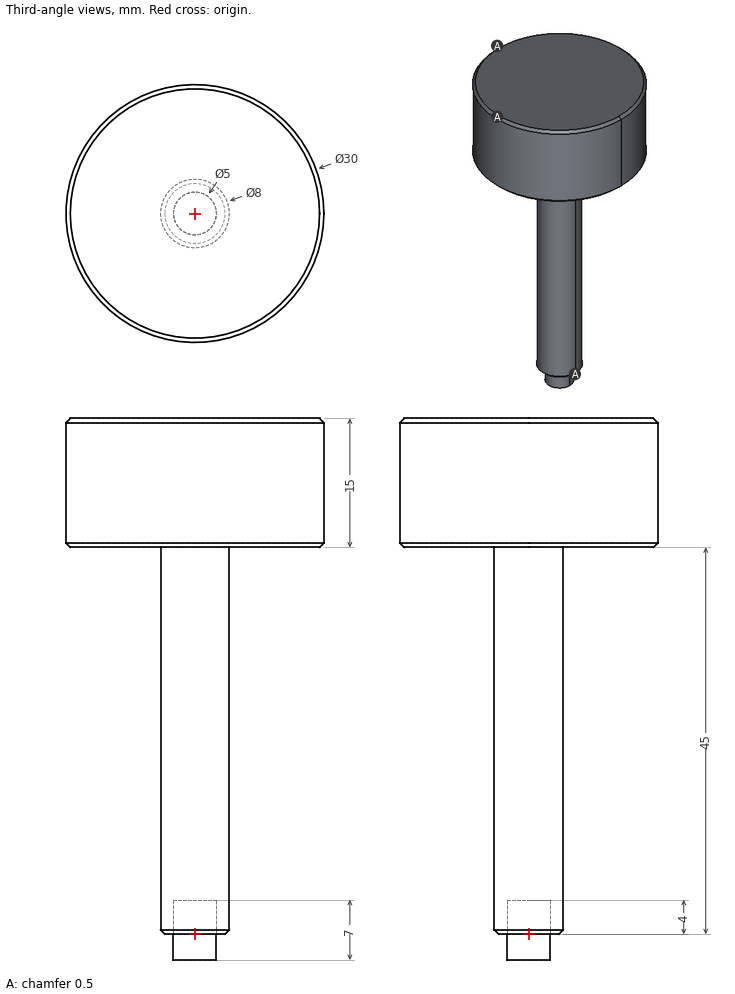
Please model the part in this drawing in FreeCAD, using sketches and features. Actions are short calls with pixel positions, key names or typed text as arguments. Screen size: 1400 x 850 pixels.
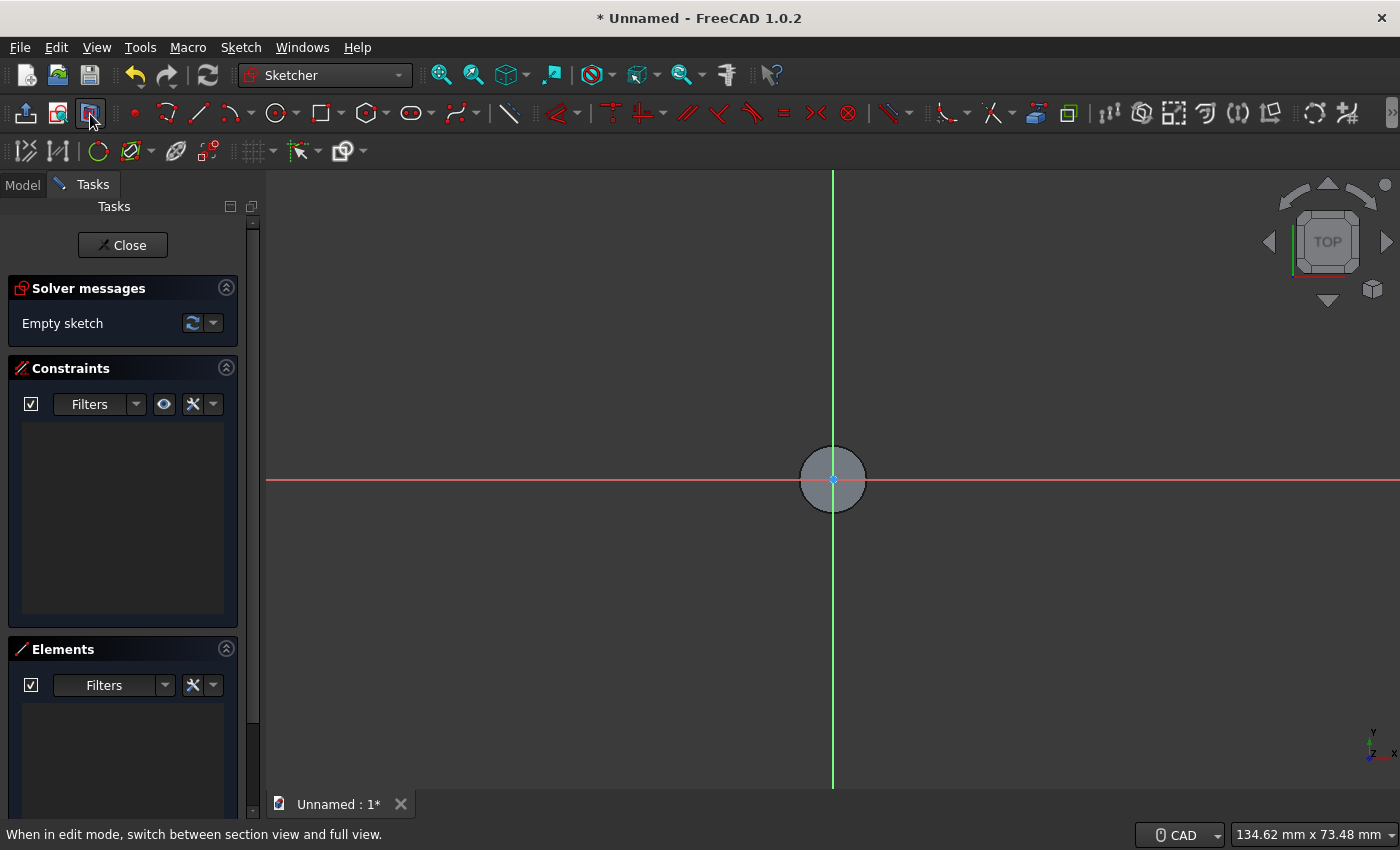
scroll(842, 479, up, 11)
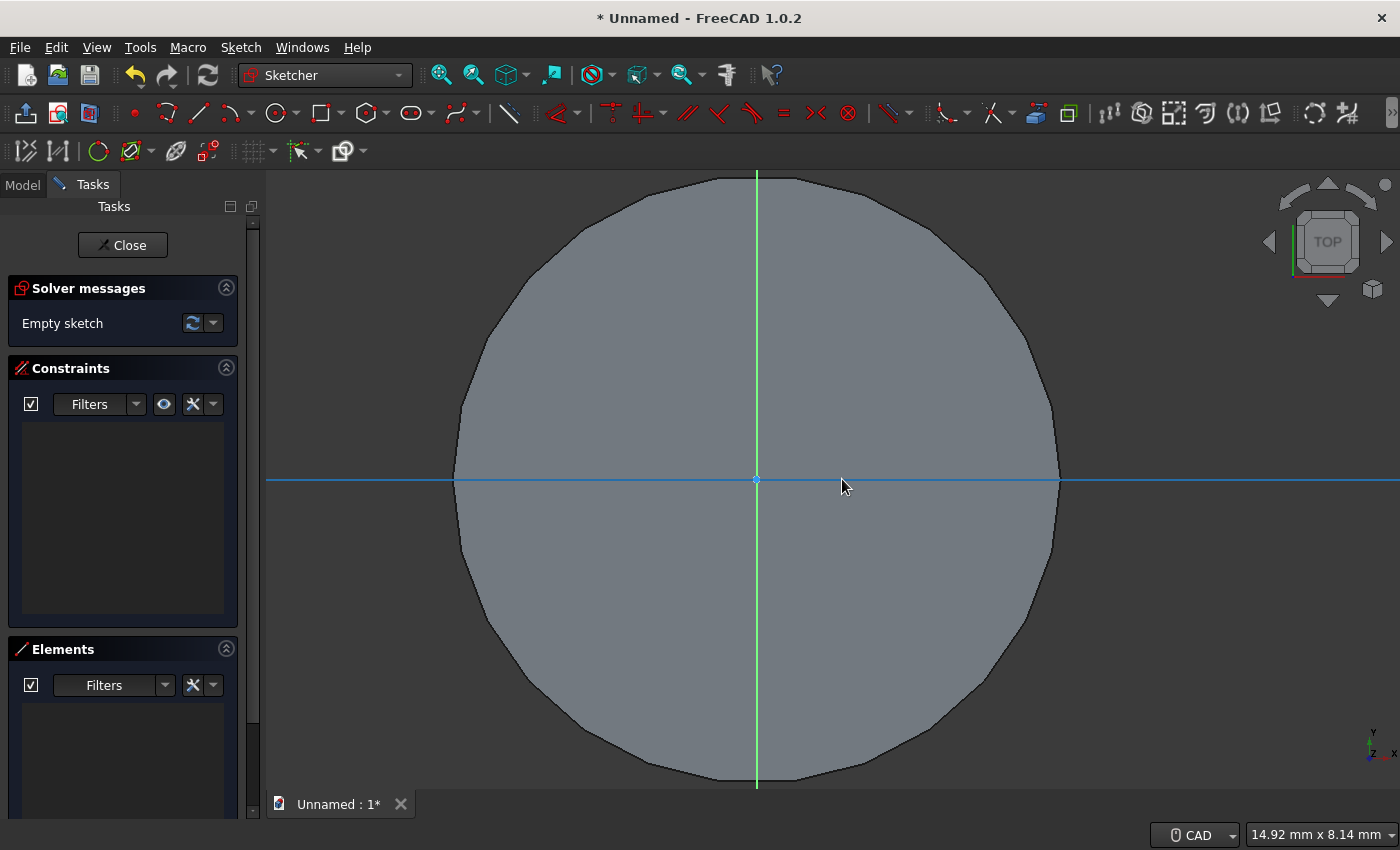
click(276, 114)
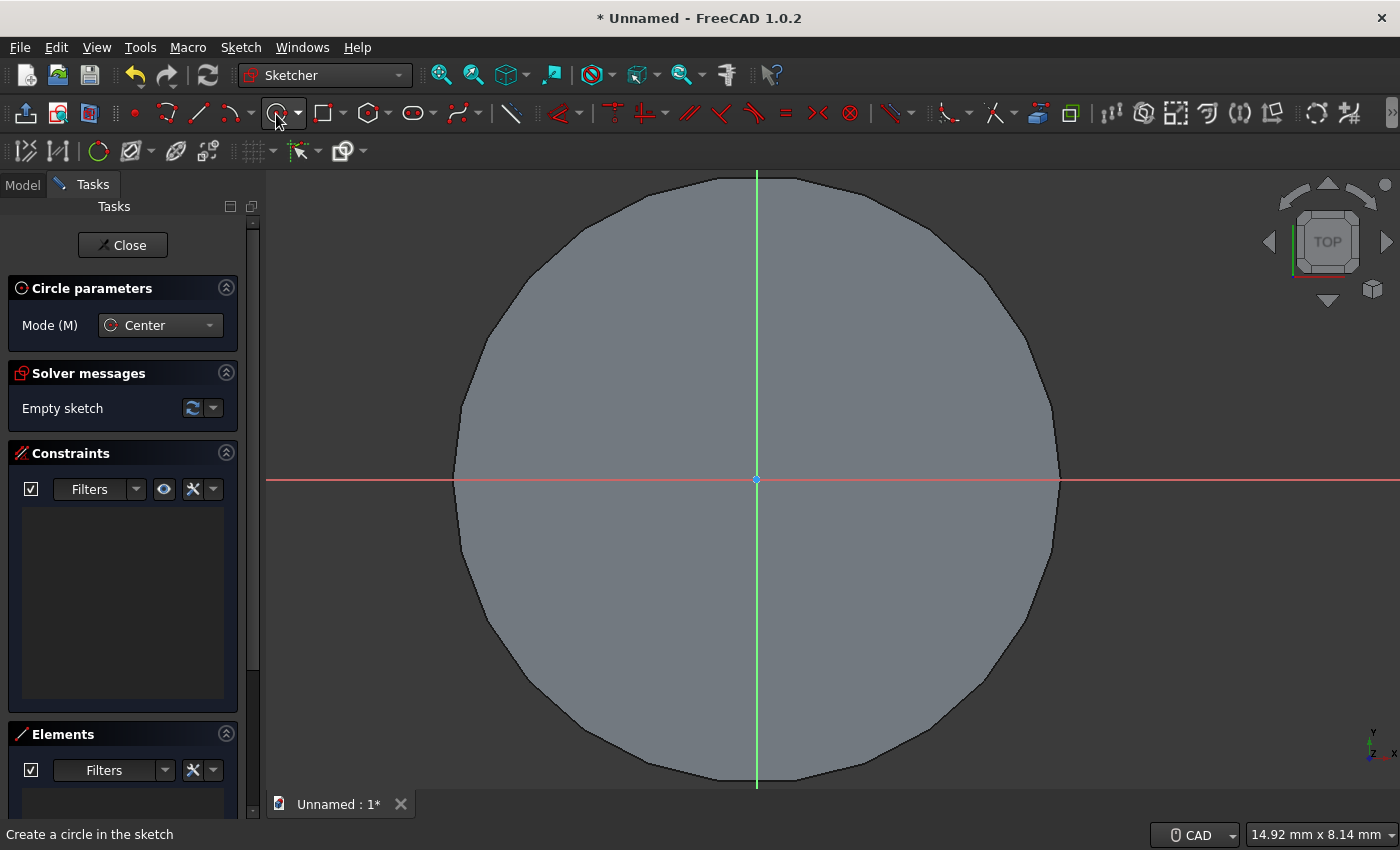
click(757, 480)
move(891, 345)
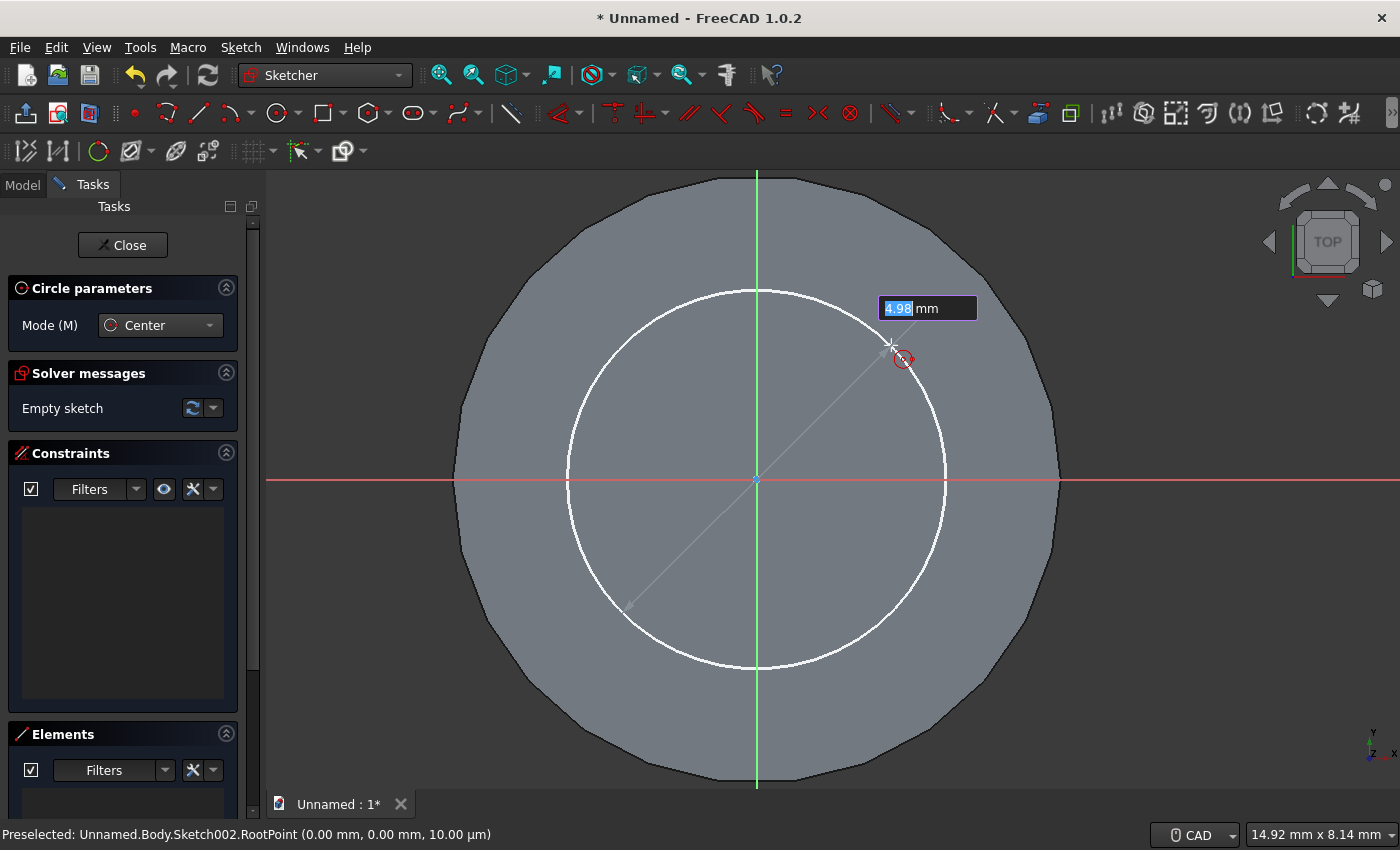
text(5)
key(Return)
key(Escape)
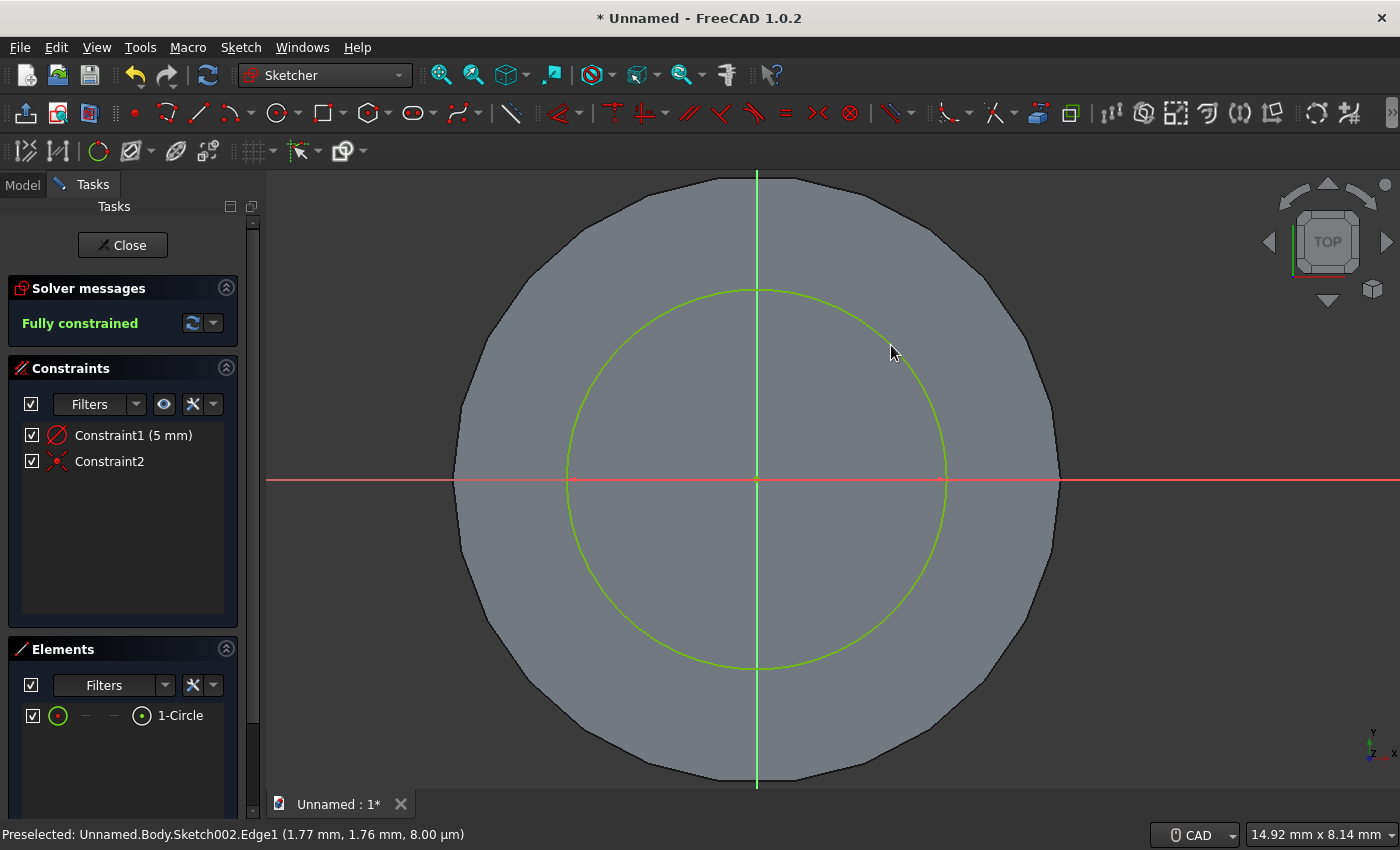
click(123, 245)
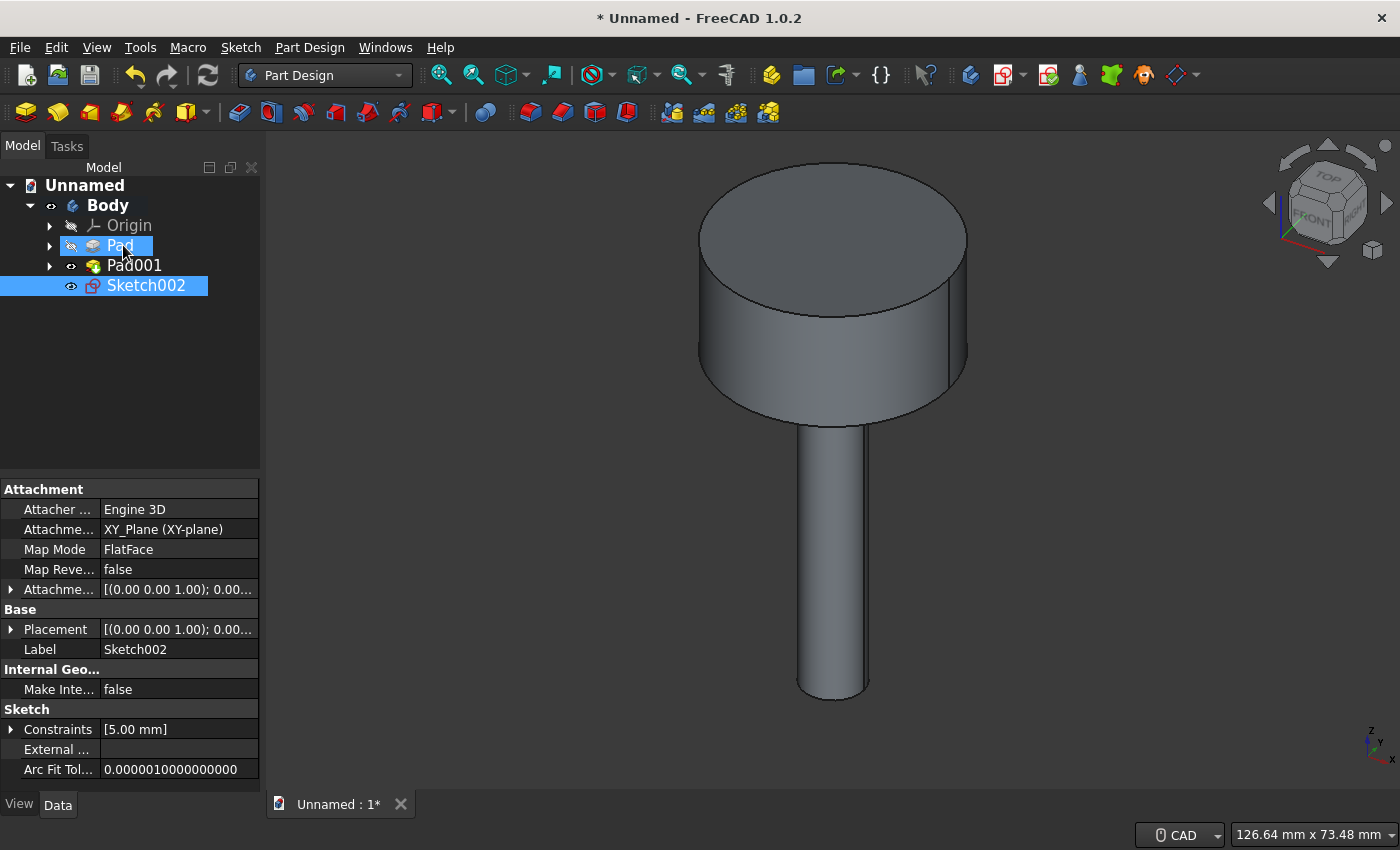
click(240, 112)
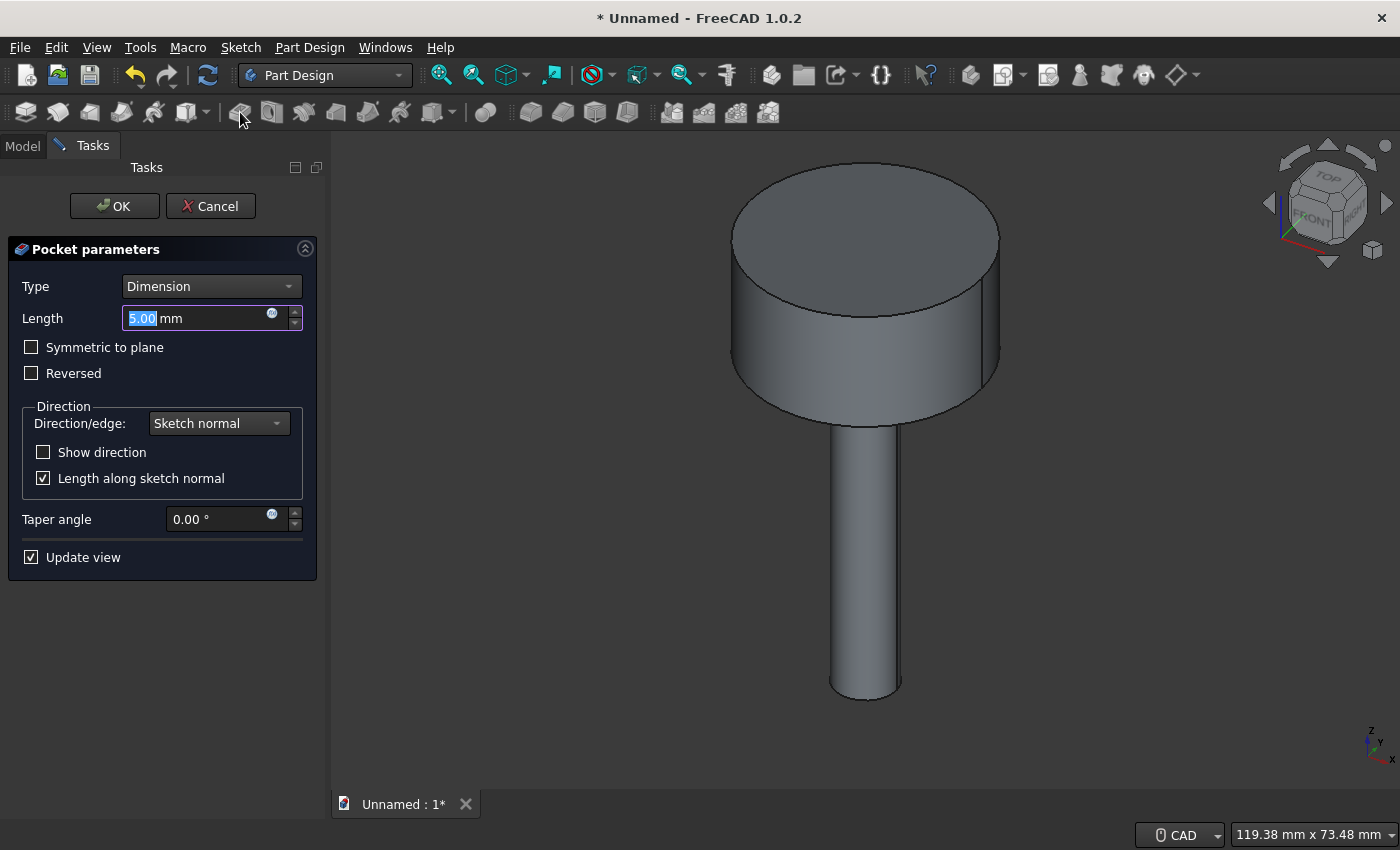
text(4)
key(Tab)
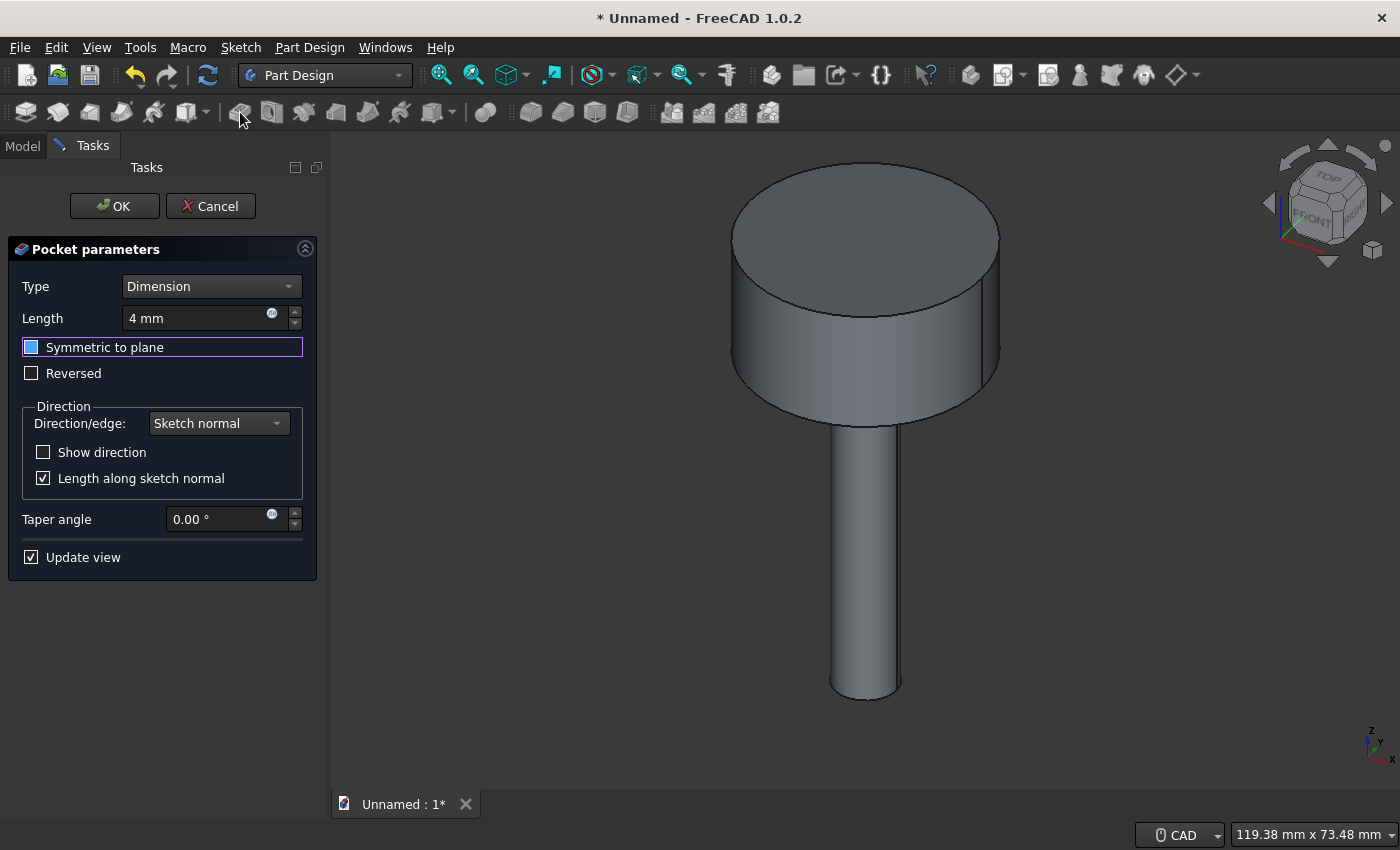
click(30, 373)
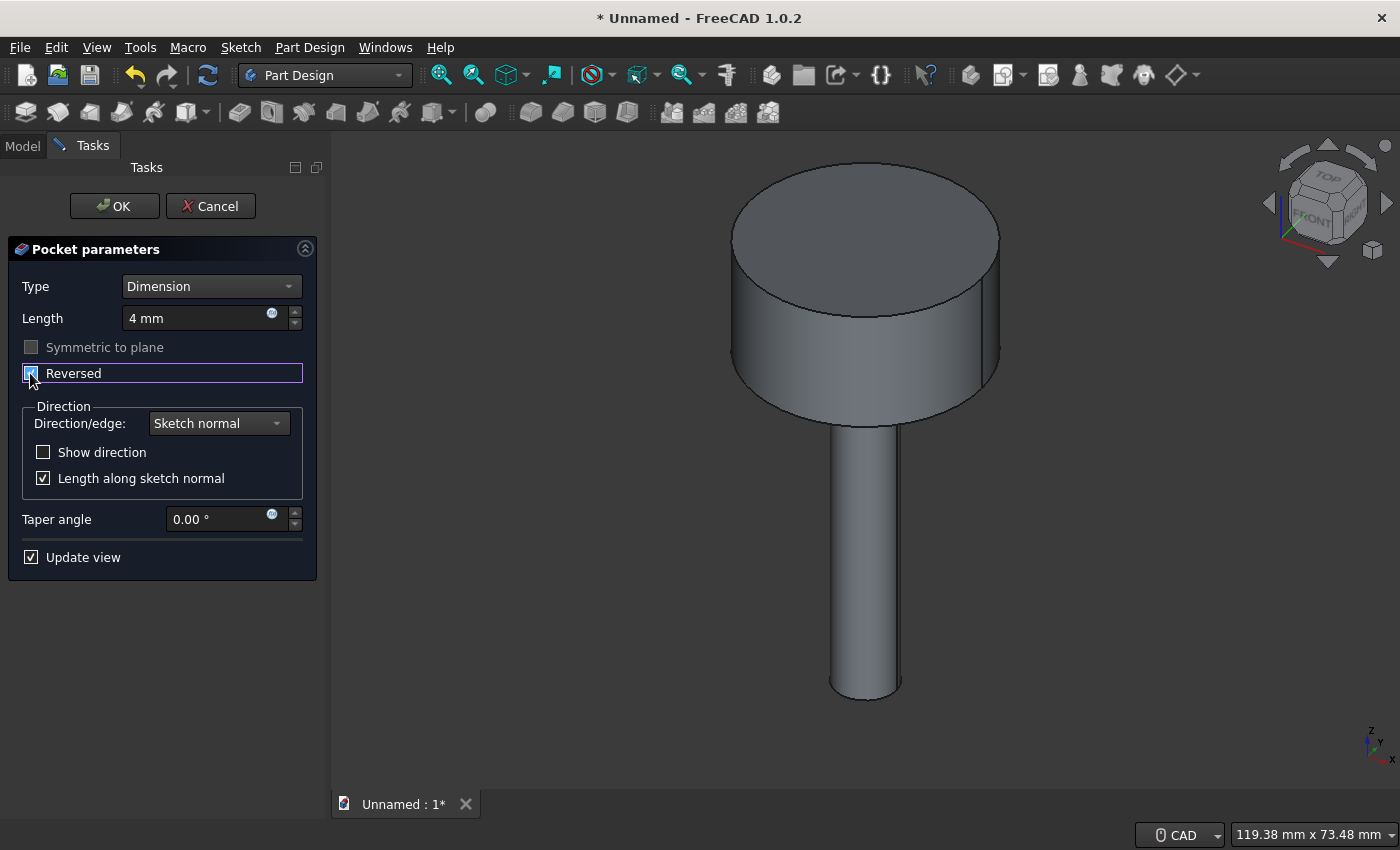
click(115, 206)